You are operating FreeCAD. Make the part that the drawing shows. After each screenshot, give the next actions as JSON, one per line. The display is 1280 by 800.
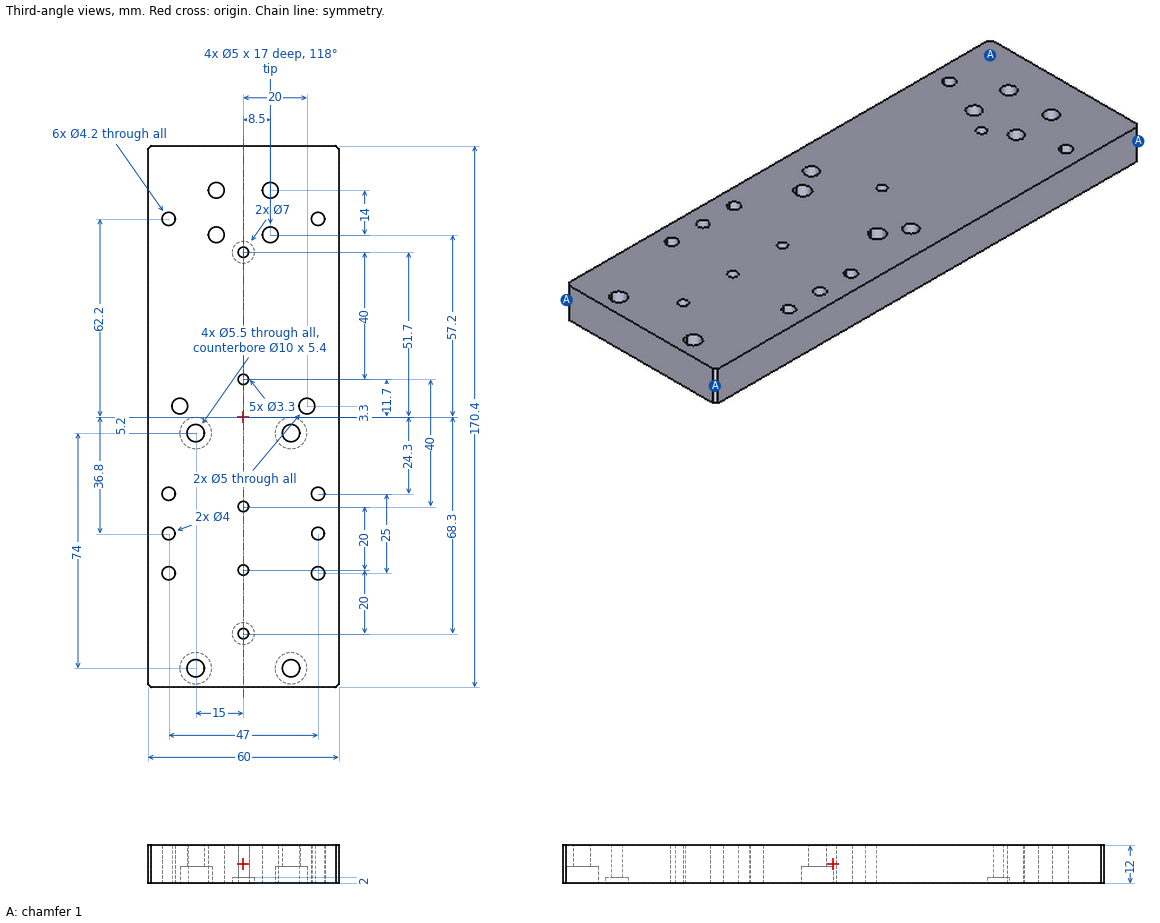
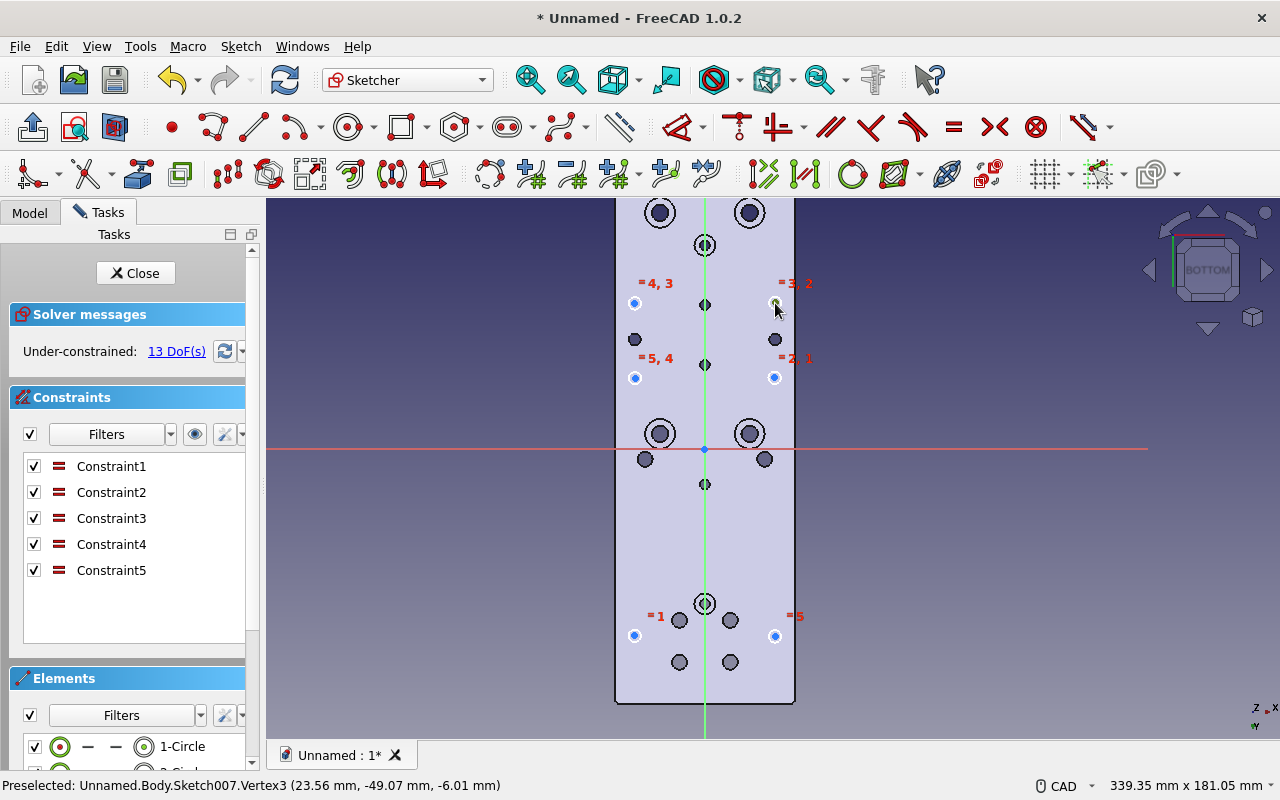
{"action": "left_click", "coordinate": [635, 303]}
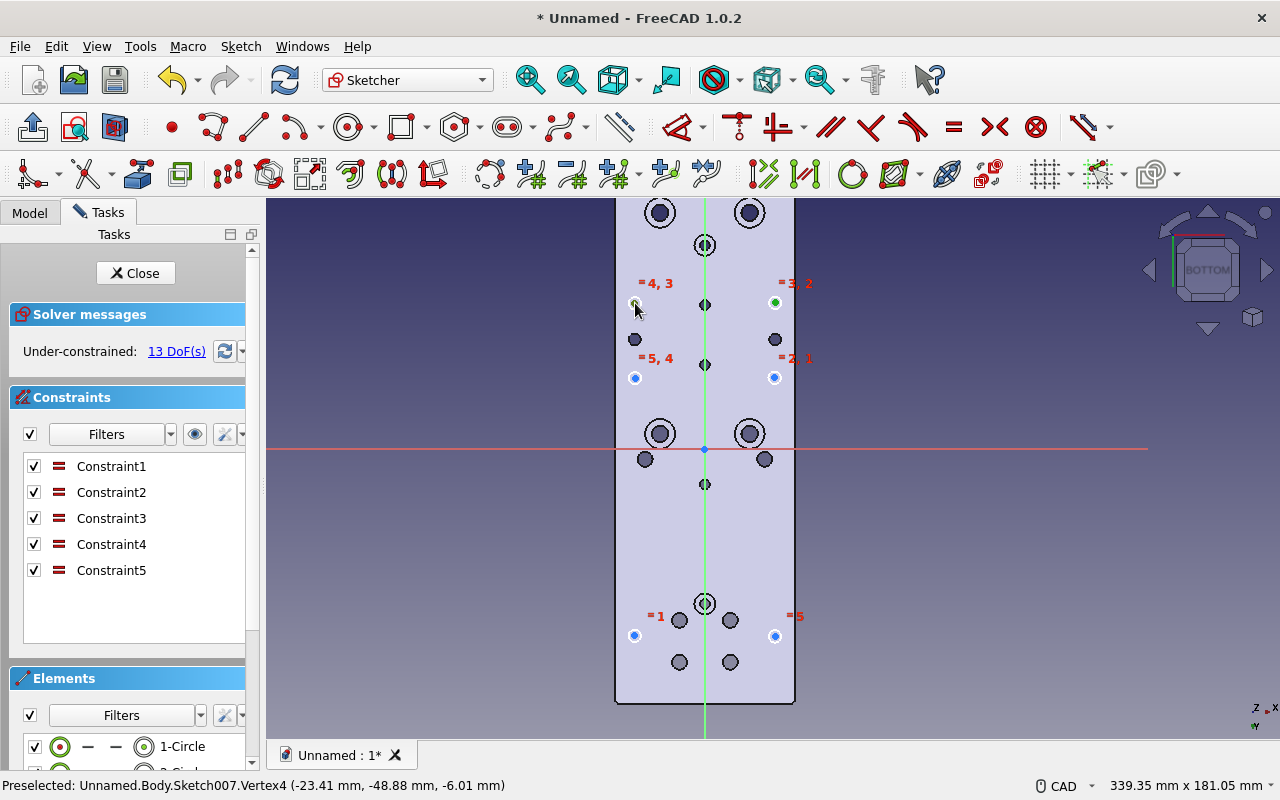
{"action": "left_click", "coordinate": [705, 676]}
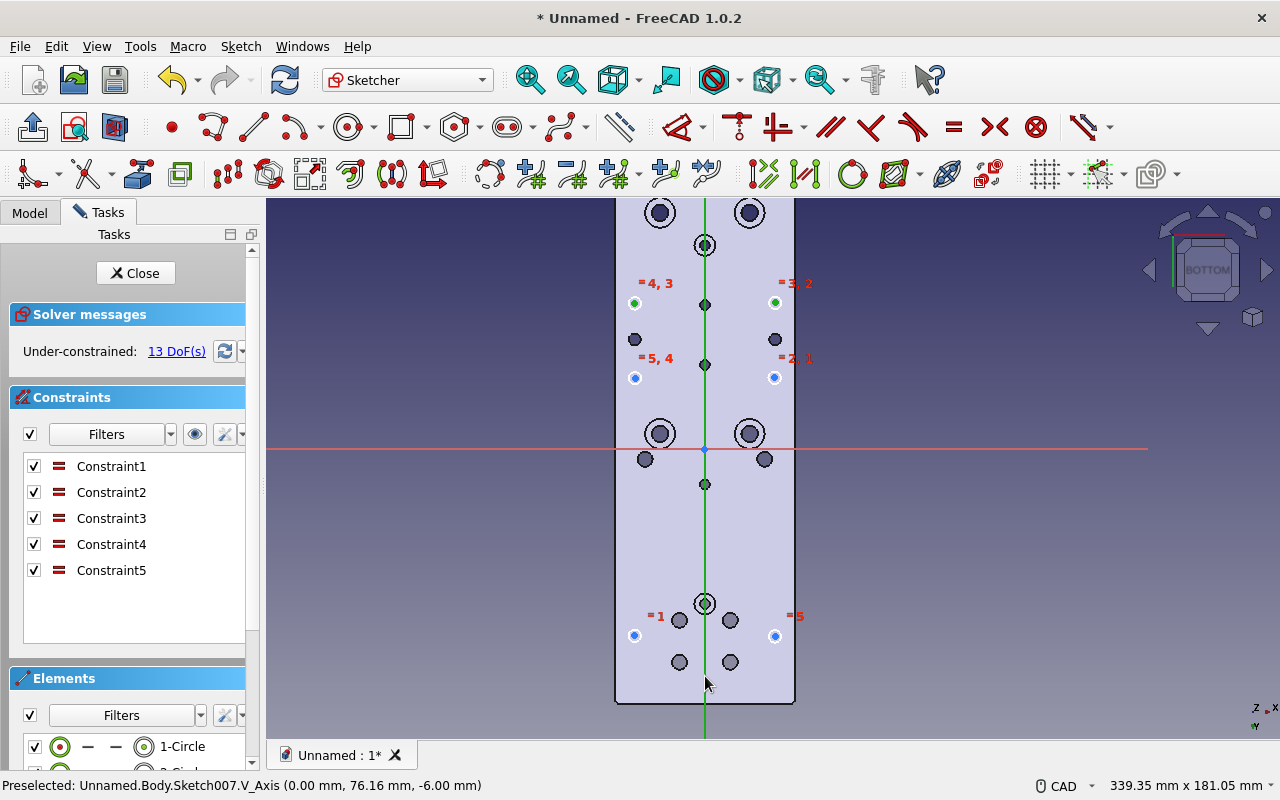
{"action": "left_click", "coordinate": [995, 128]}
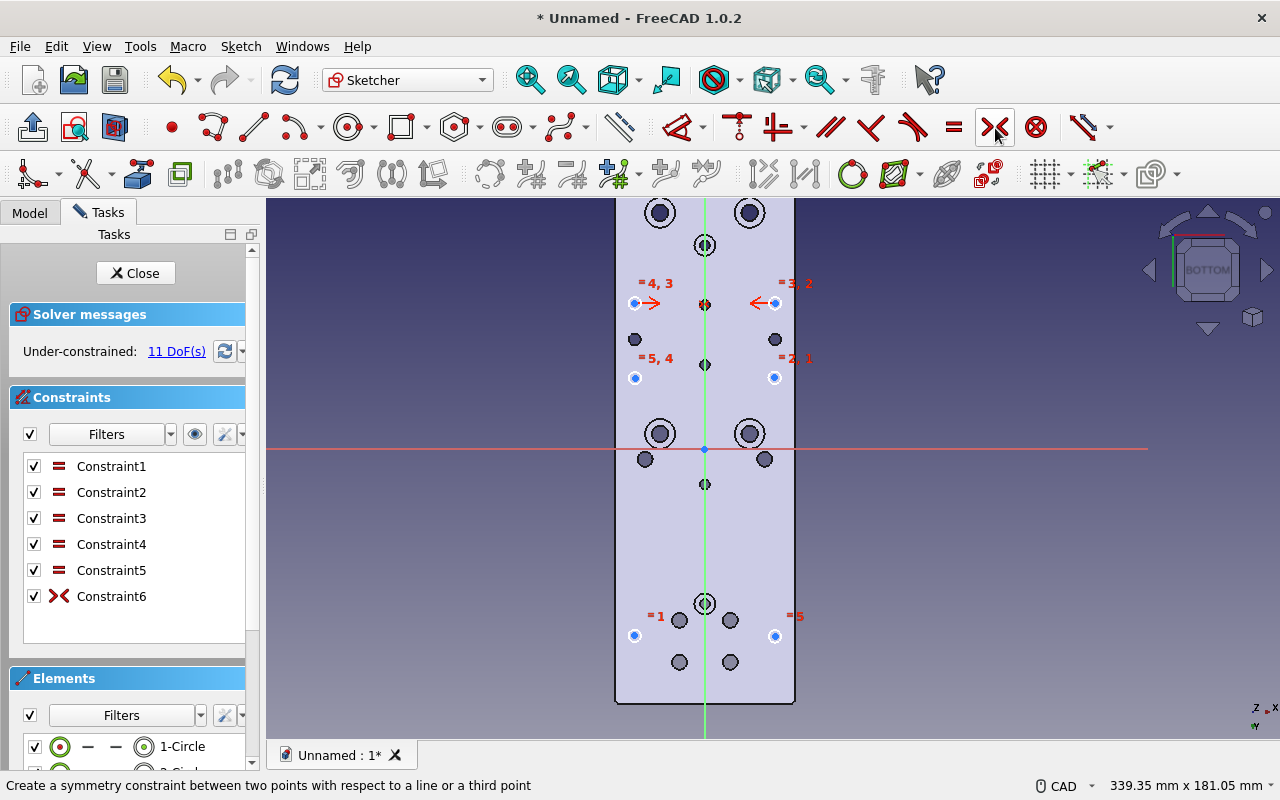
{"action": "left_click", "coordinate": [775, 378]}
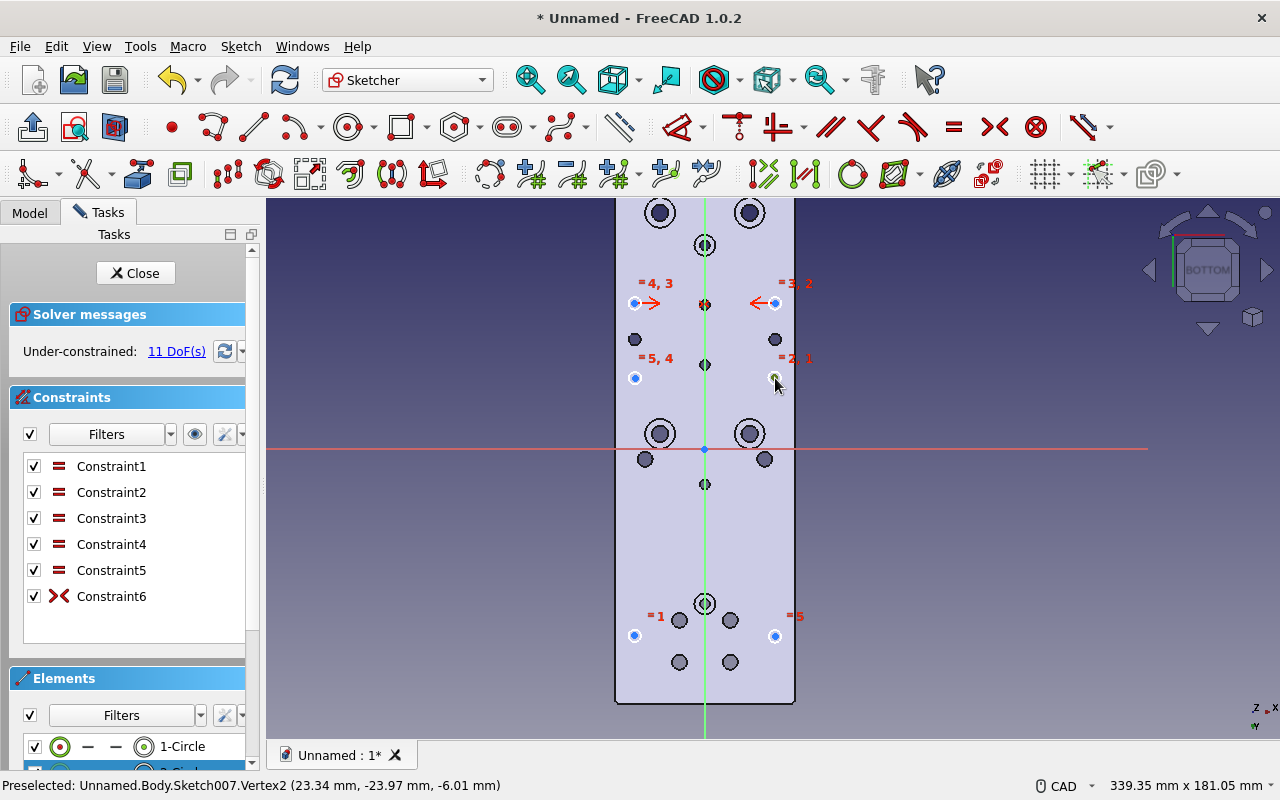
{"action": "left_click", "coordinate": [635, 378]}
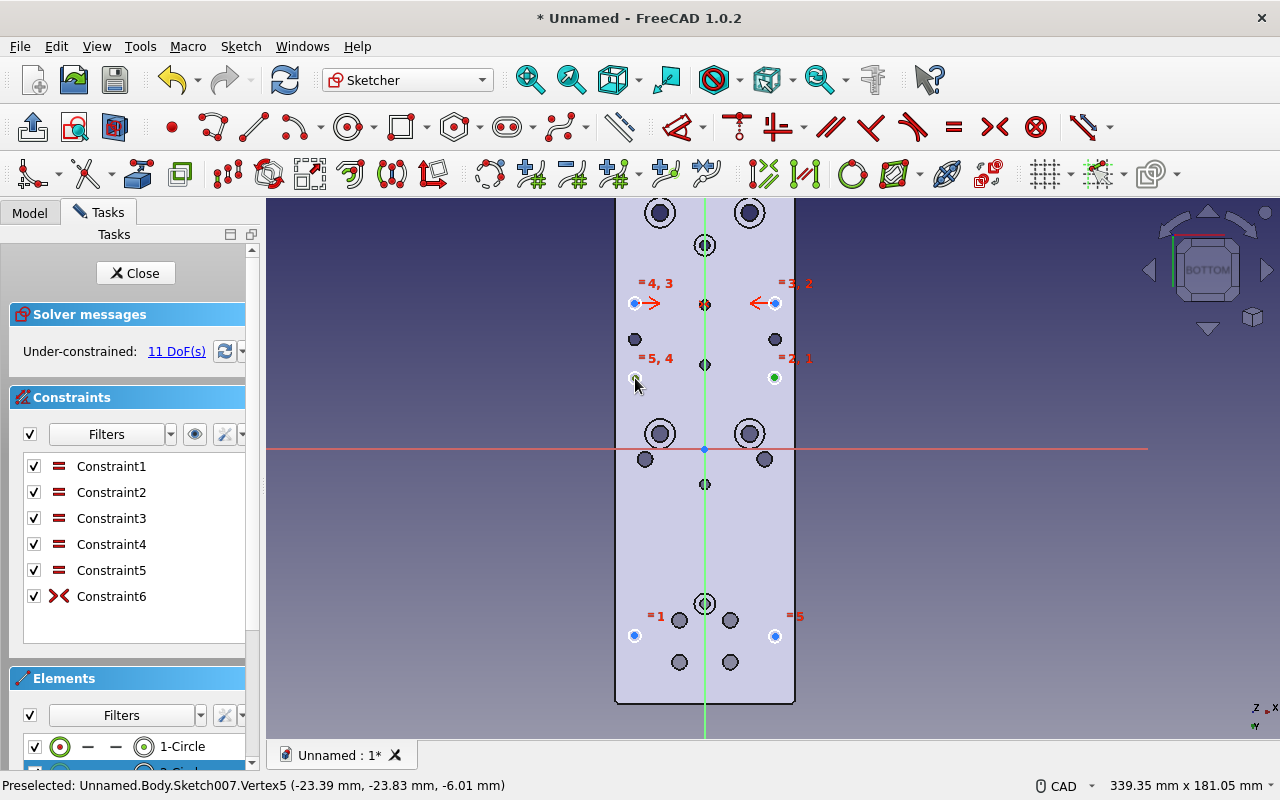
{"action": "left_click", "coordinate": [705, 676]}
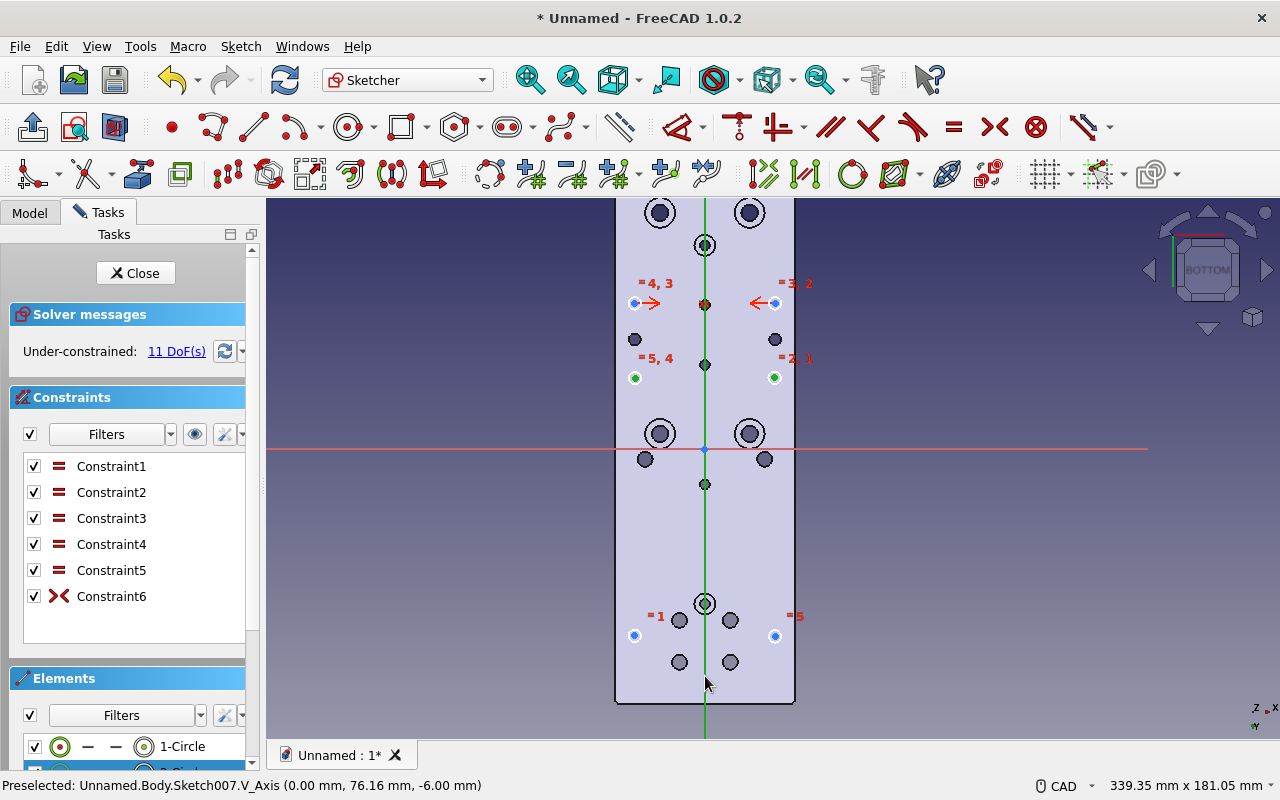
{"action": "left_click", "coordinate": [995, 128]}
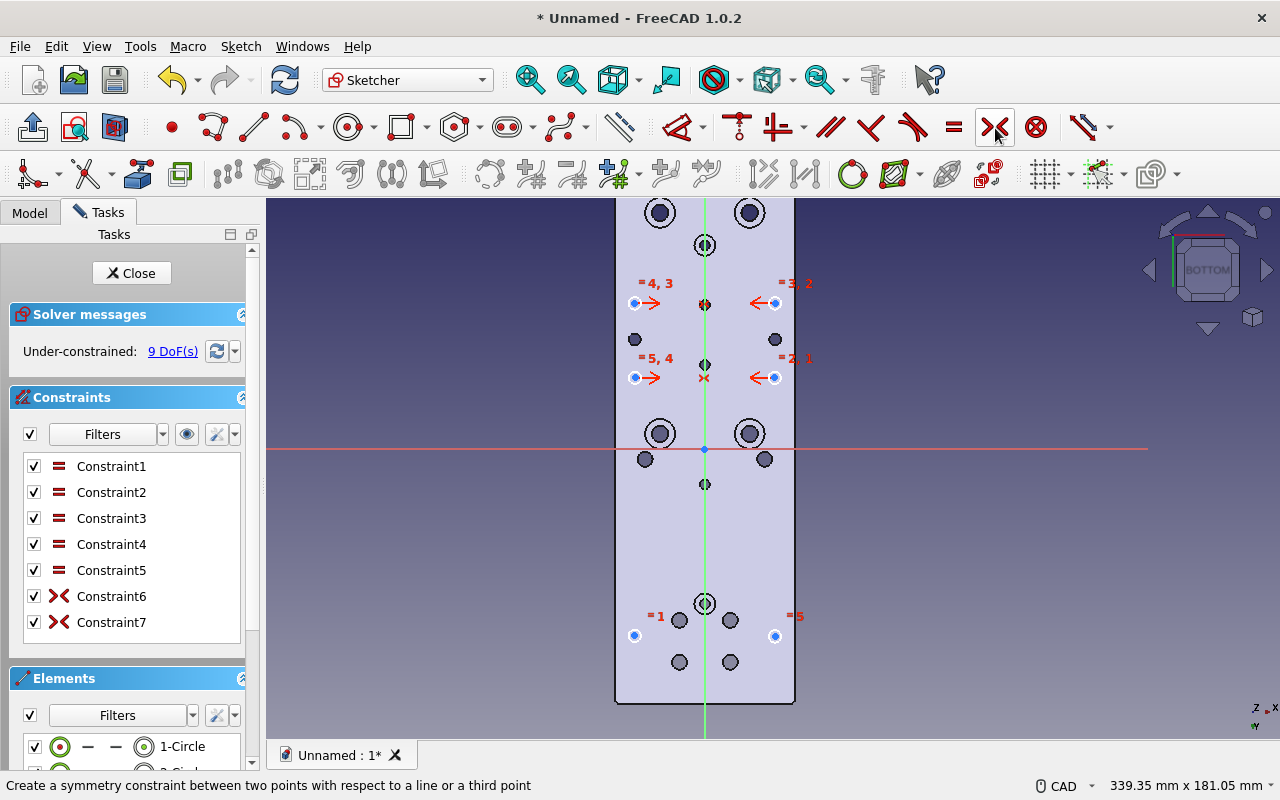
{"action": "left_click", "coordinate": [635, 636]}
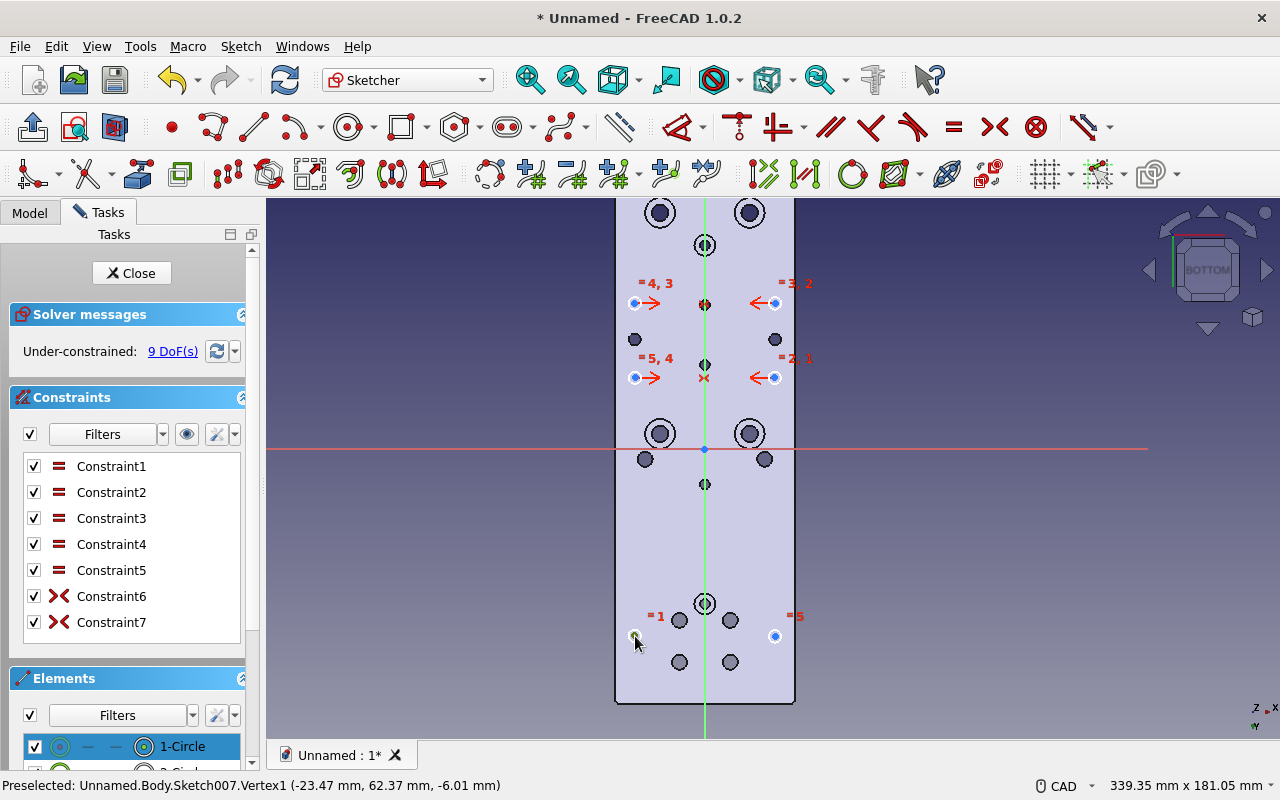
{"action": "left_click", "coordinate": [775, 636]}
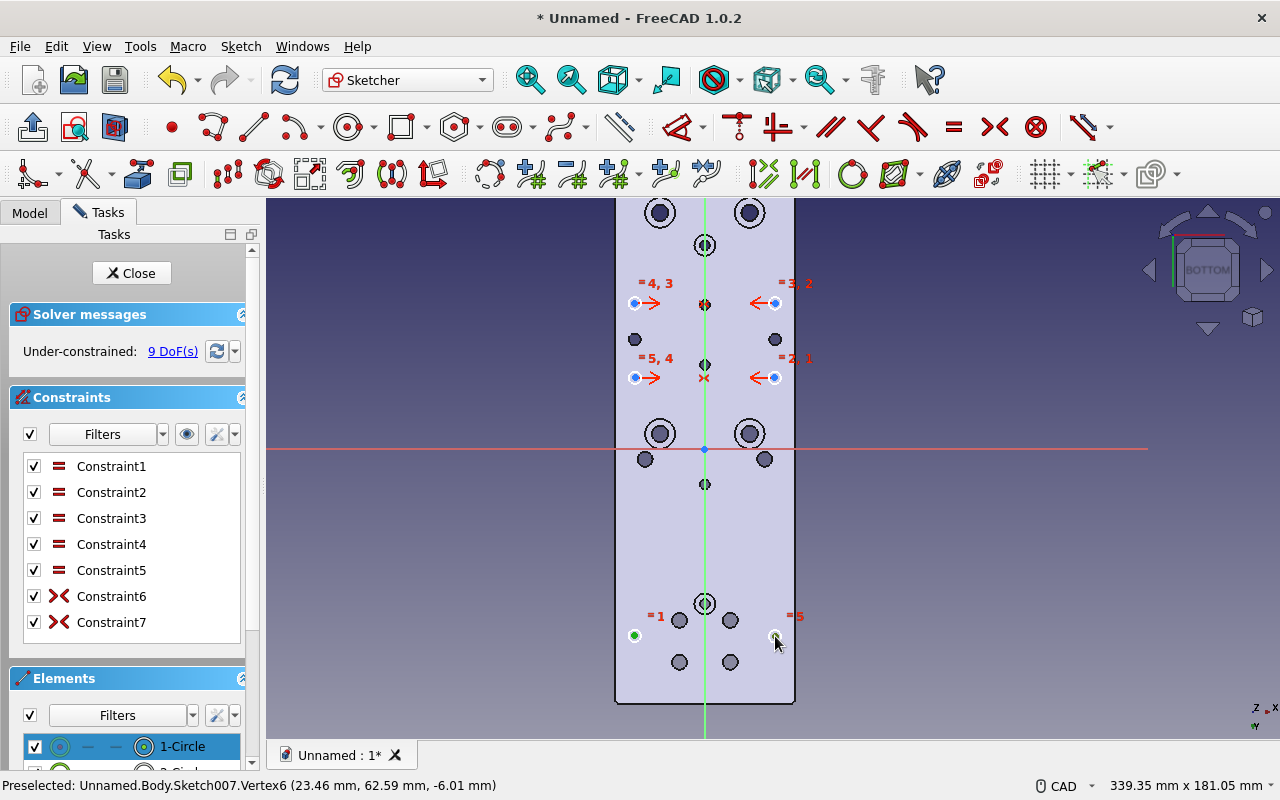
{"action": "left_click", "coordinate": [705, 676]}